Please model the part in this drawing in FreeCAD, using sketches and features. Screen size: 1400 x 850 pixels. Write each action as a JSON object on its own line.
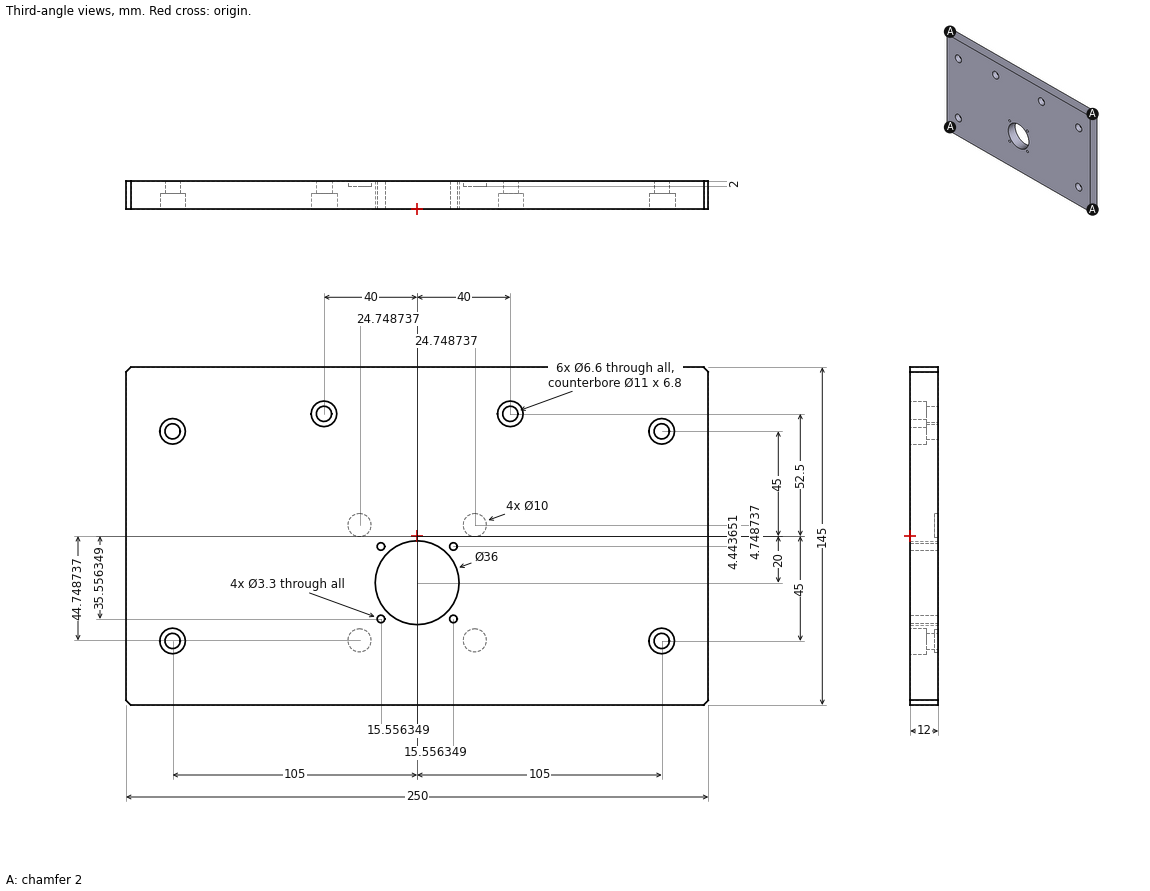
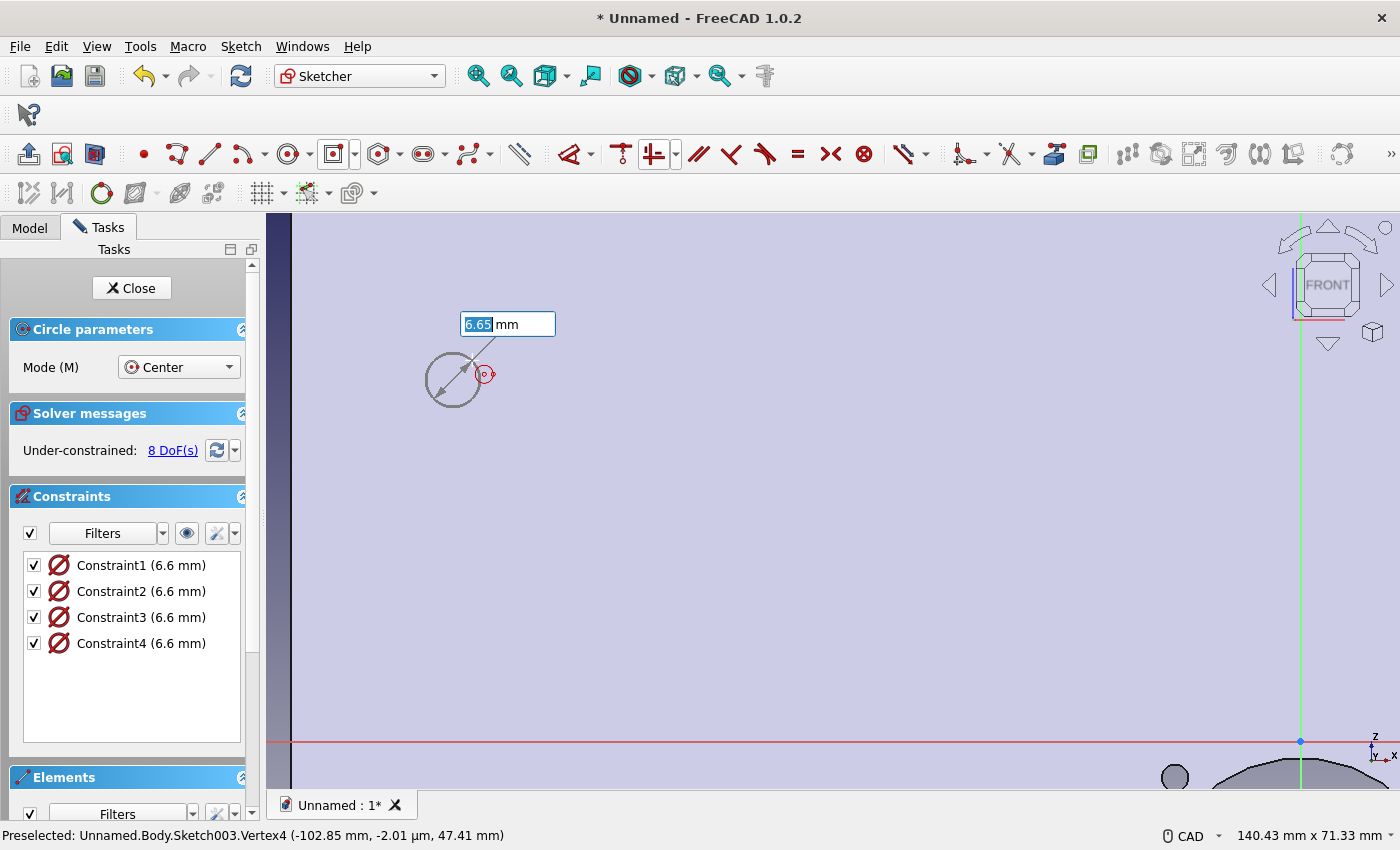
{"action": "type", "text": "6.6"}
{"action": "key", "text": "Return"}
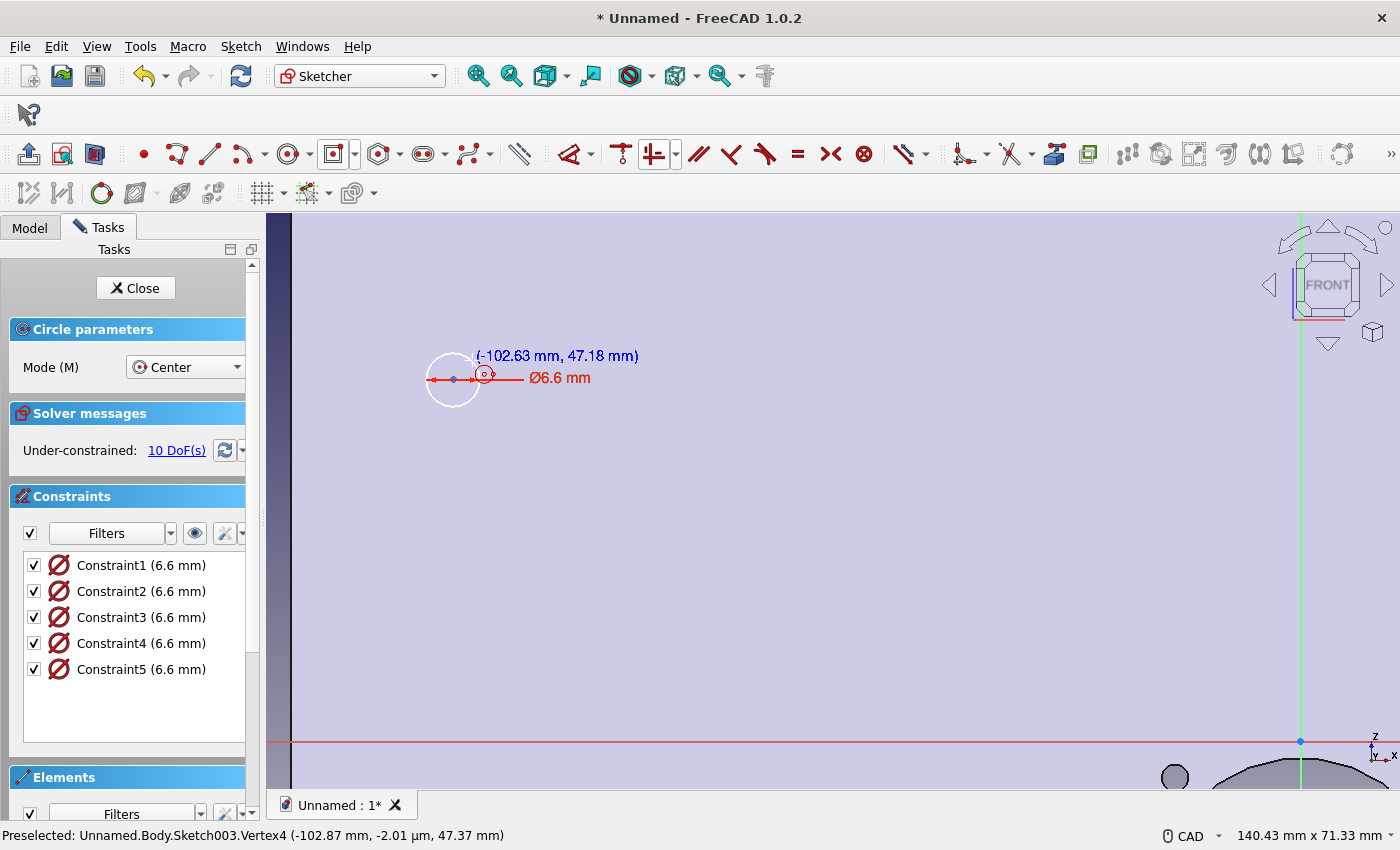
{"action": "left_click", "coordinate": [978, 318]}
{"action": "mouse_move", "coordinate": [997, 299]}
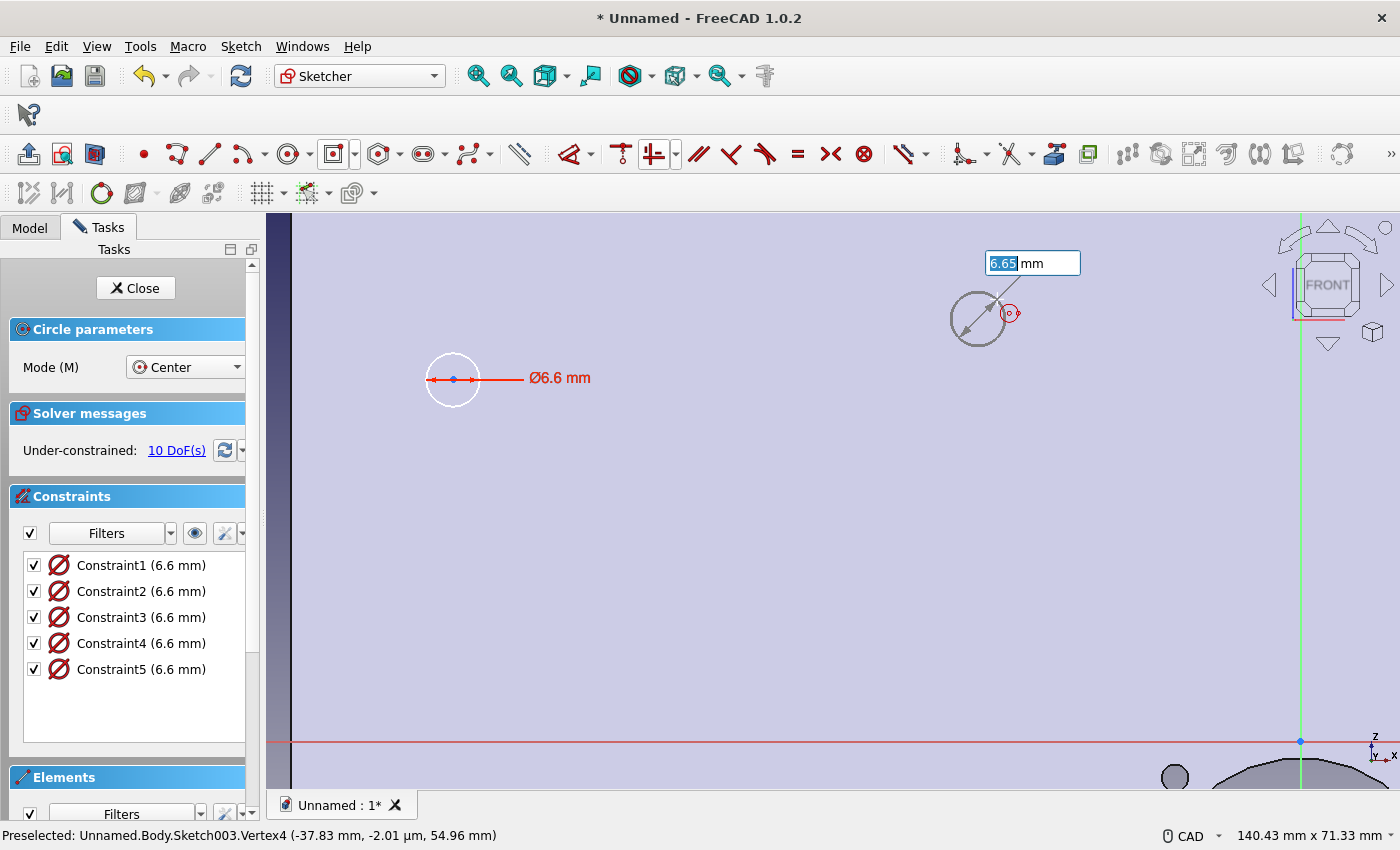
{"action": "type", "text": "6.6"}
{"action": "key", "text": "Return"}
{"action": "key", "text": "Escape"}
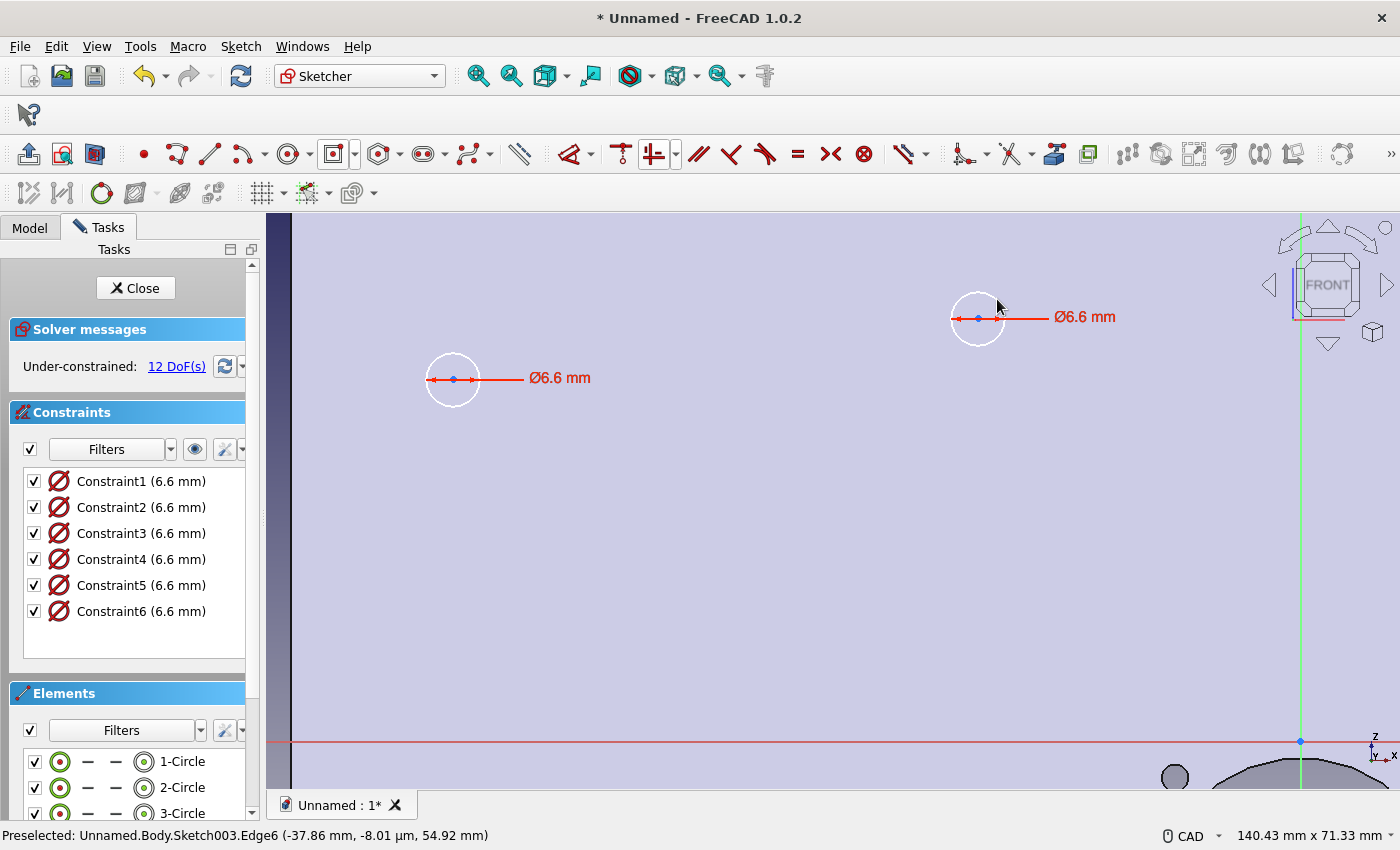
{"action": "scroll", "coordinate": [452, 378], "scroll_direction": "down", "scroll_amount": 5}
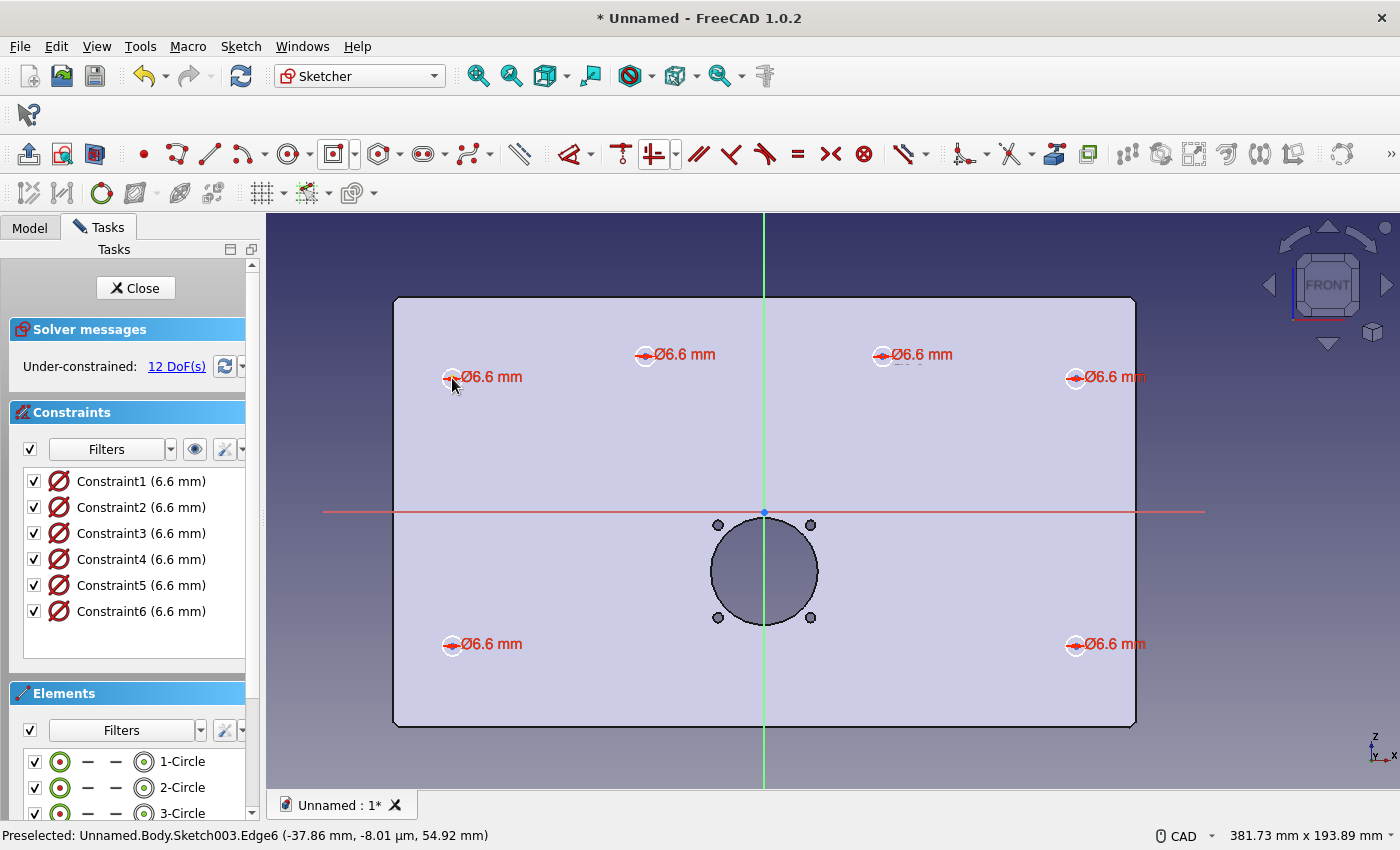
{"action": "left_click", "coordinate": [1076, 646]}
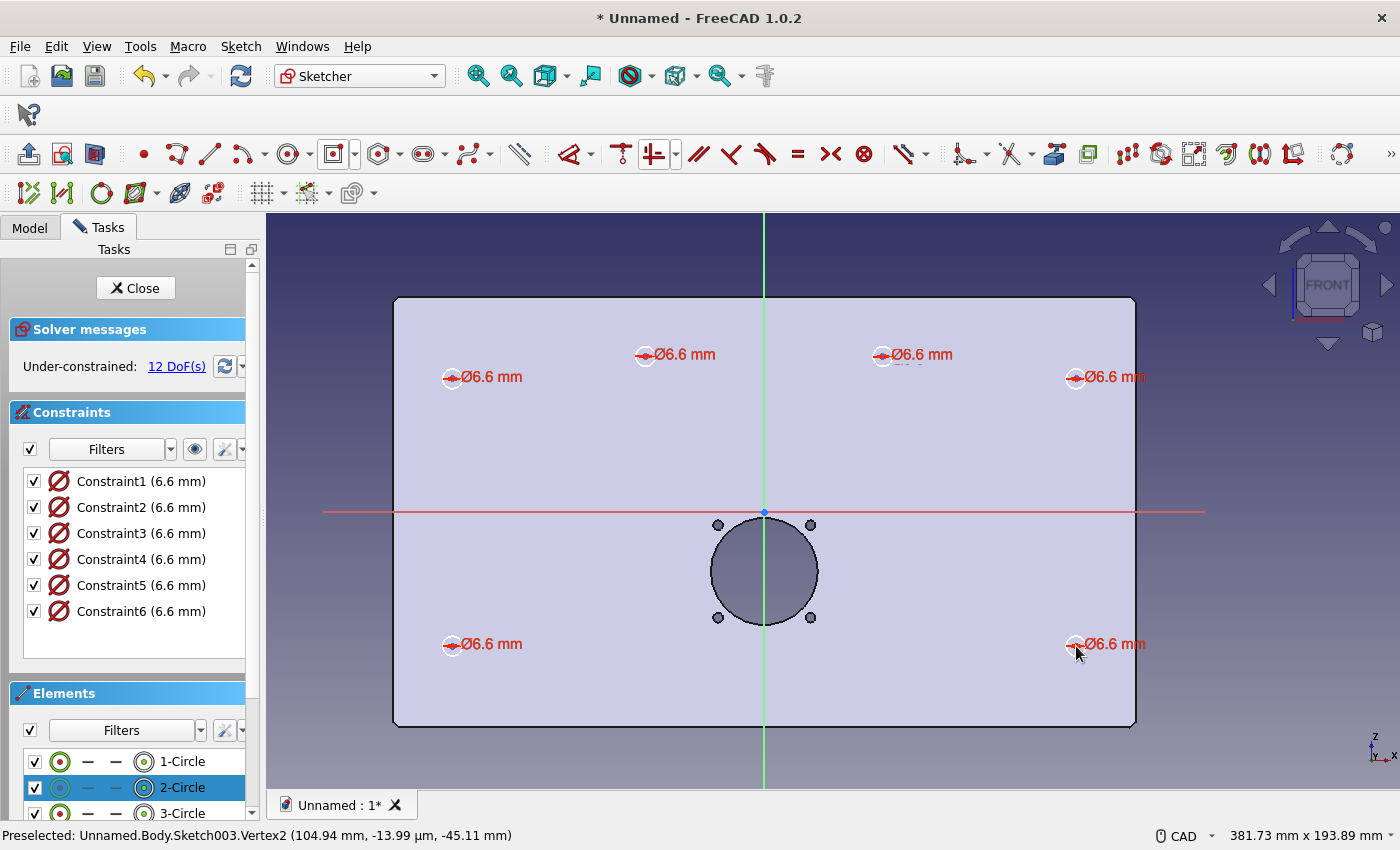
{"action": "left_click", "coordinate": [1076, 379]}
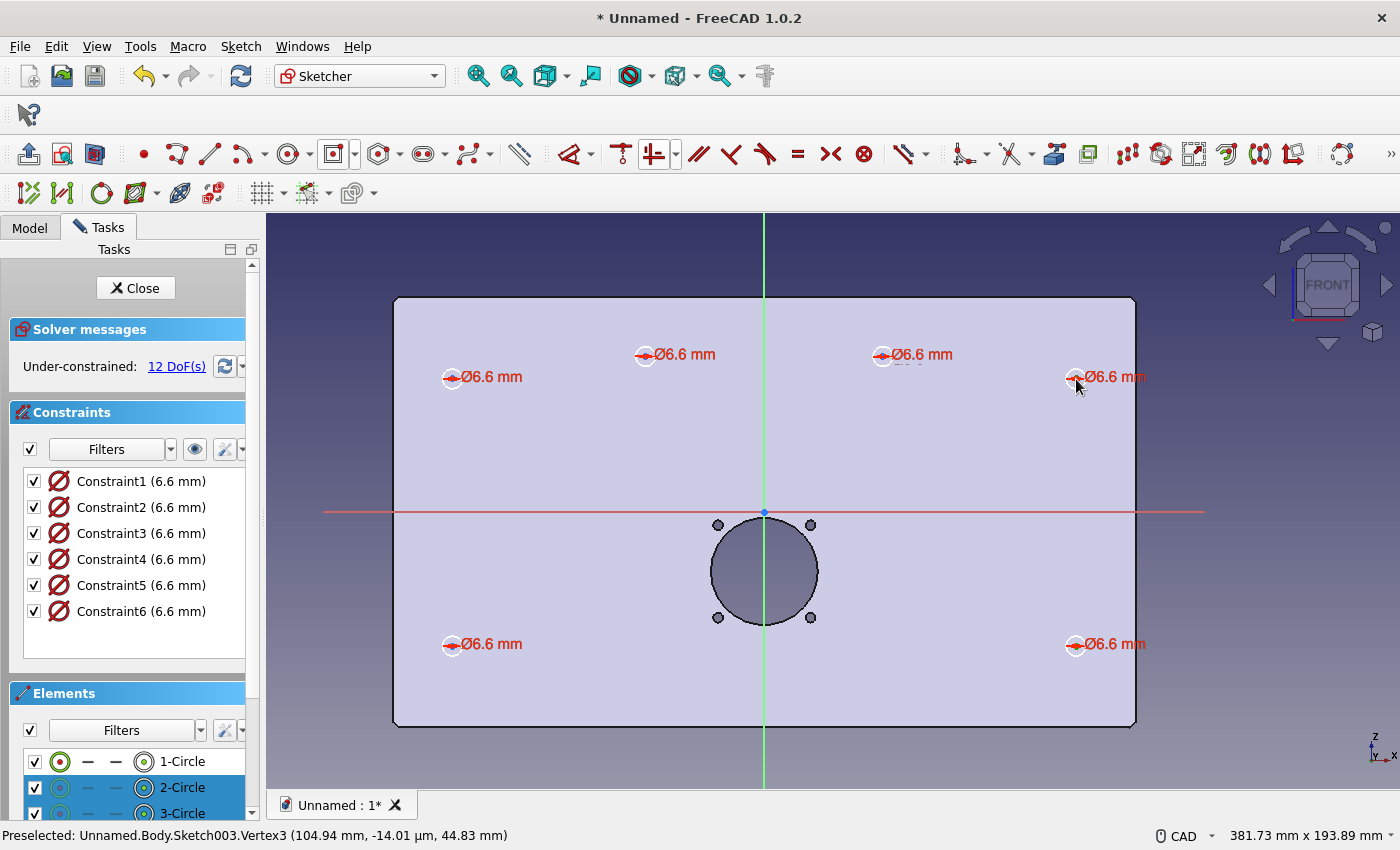
{"action": "key", "text": "v"}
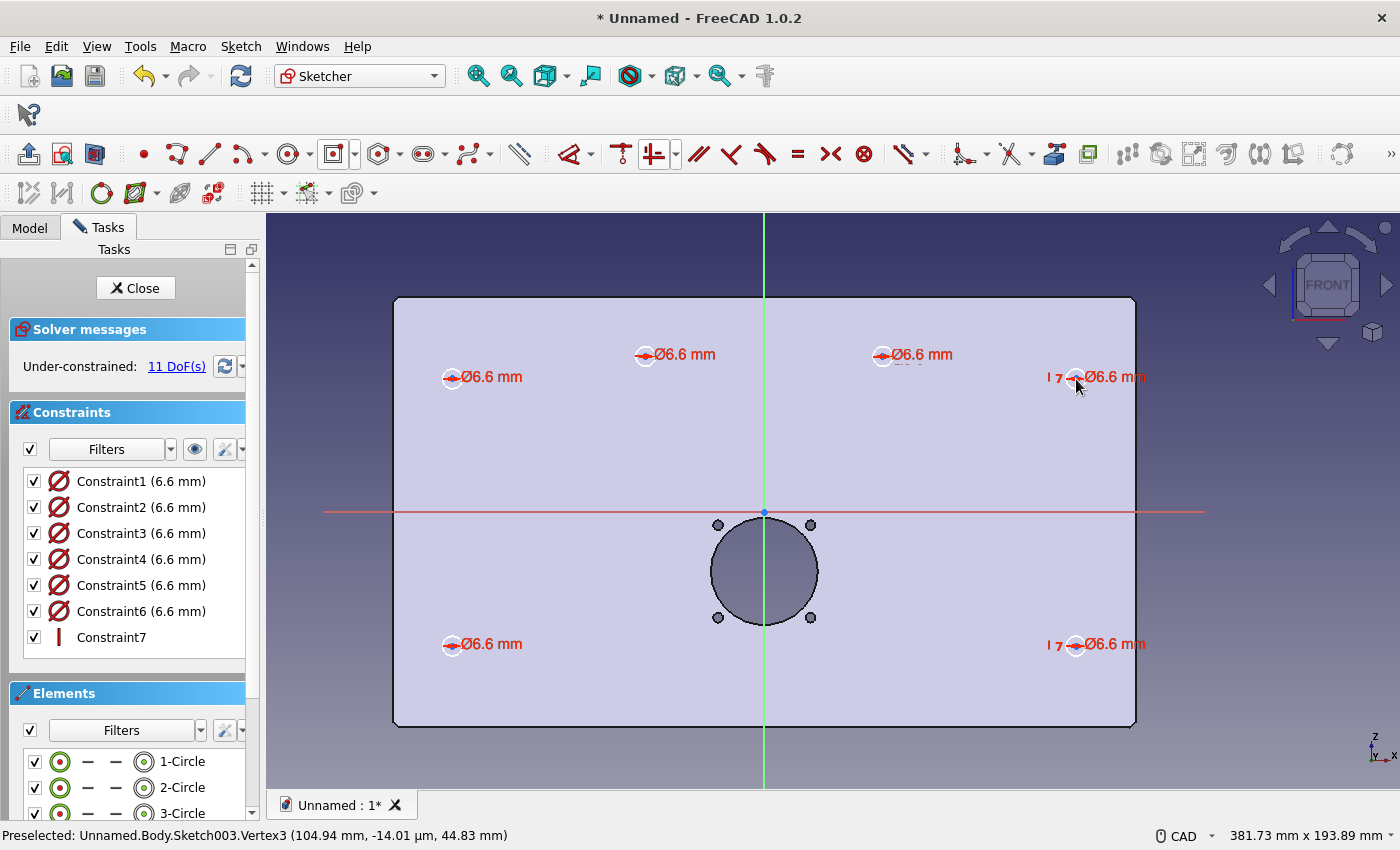
{"action": "left_click", "coordinate": [1076, 646]}